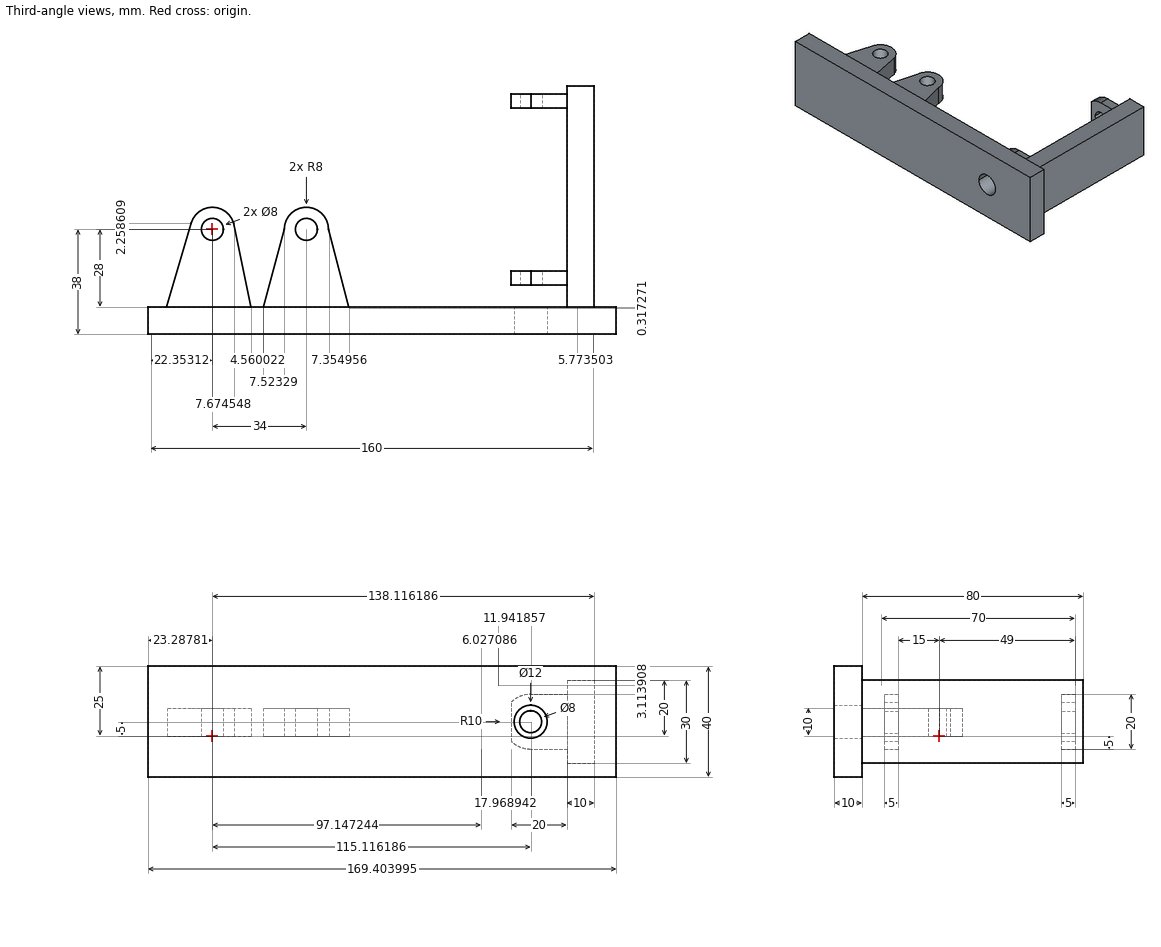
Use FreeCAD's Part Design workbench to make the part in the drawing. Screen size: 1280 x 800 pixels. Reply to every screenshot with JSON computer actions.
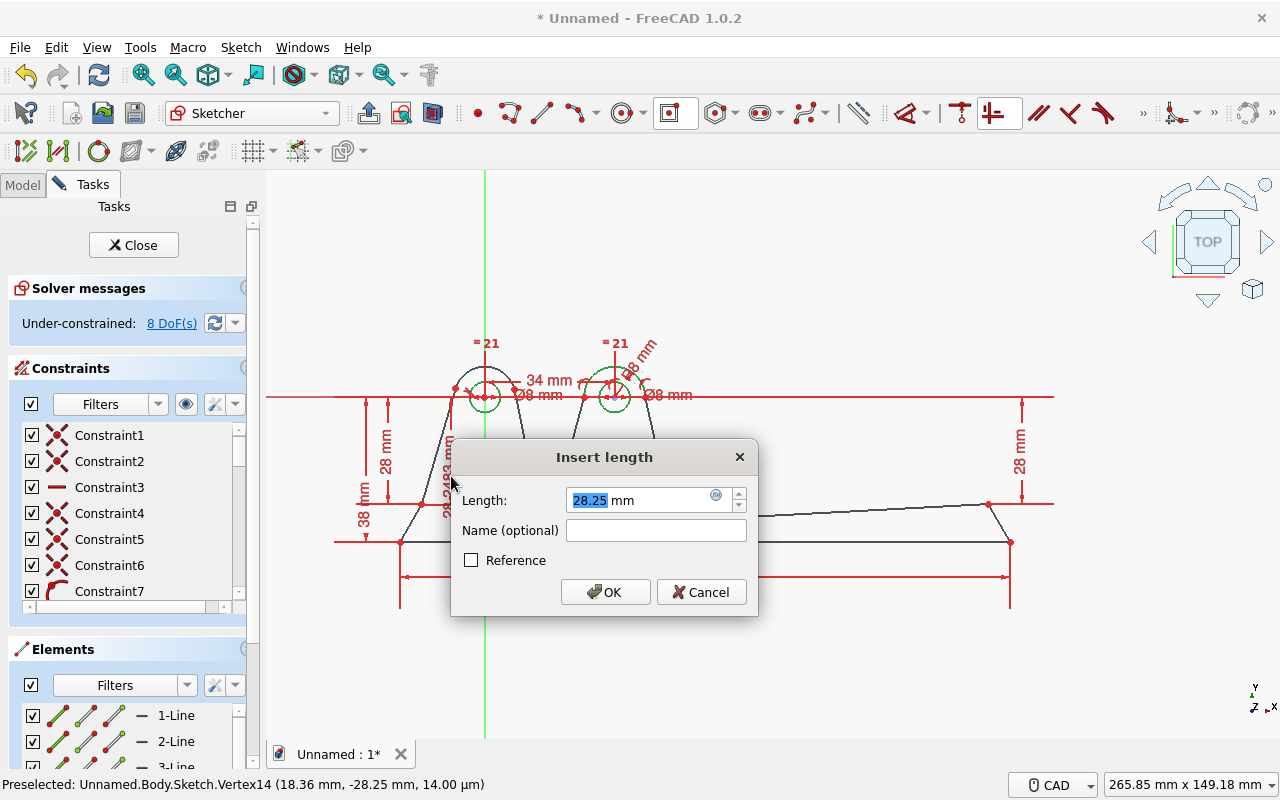
{"action": "type", "text": "28"}
{"action": "key", "text": "Return"}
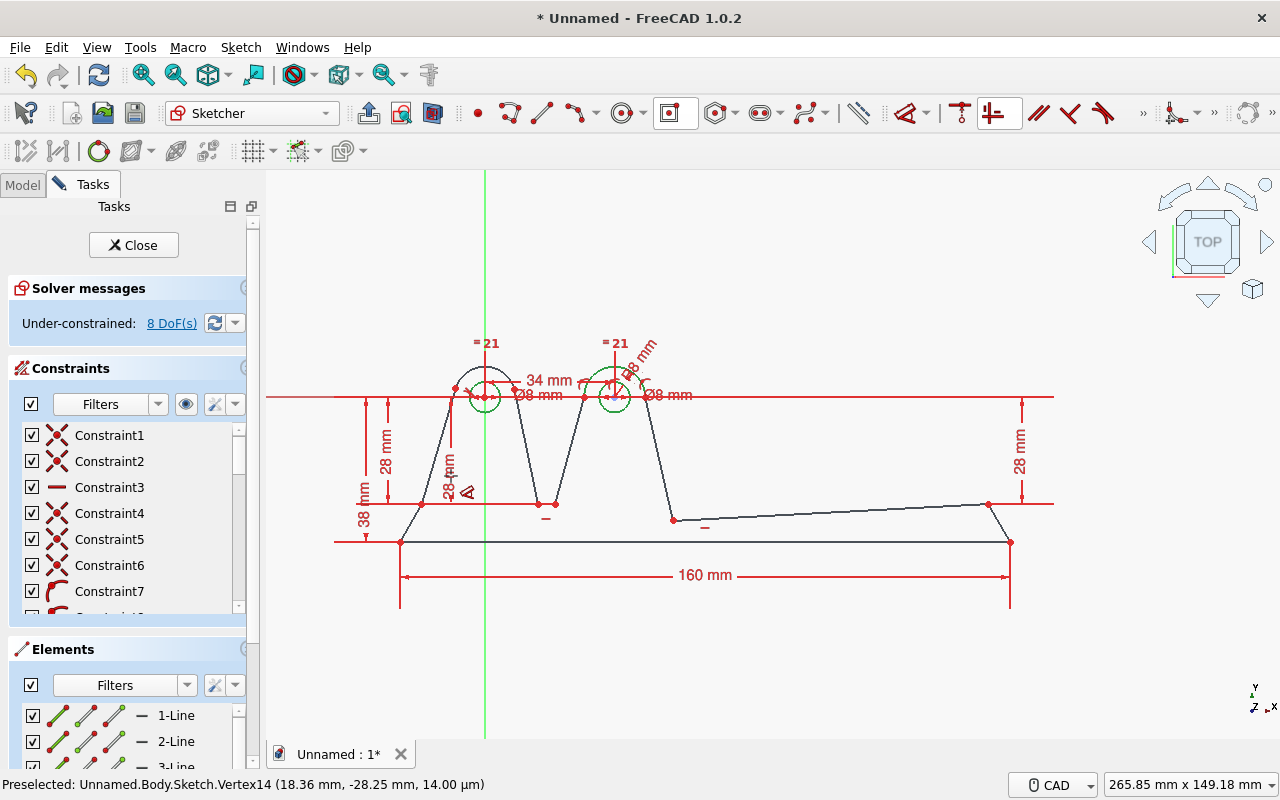
{"action": "scroll", "coordinate": [546, 504], "scroll_direction": "up", "scroll_amount": 5}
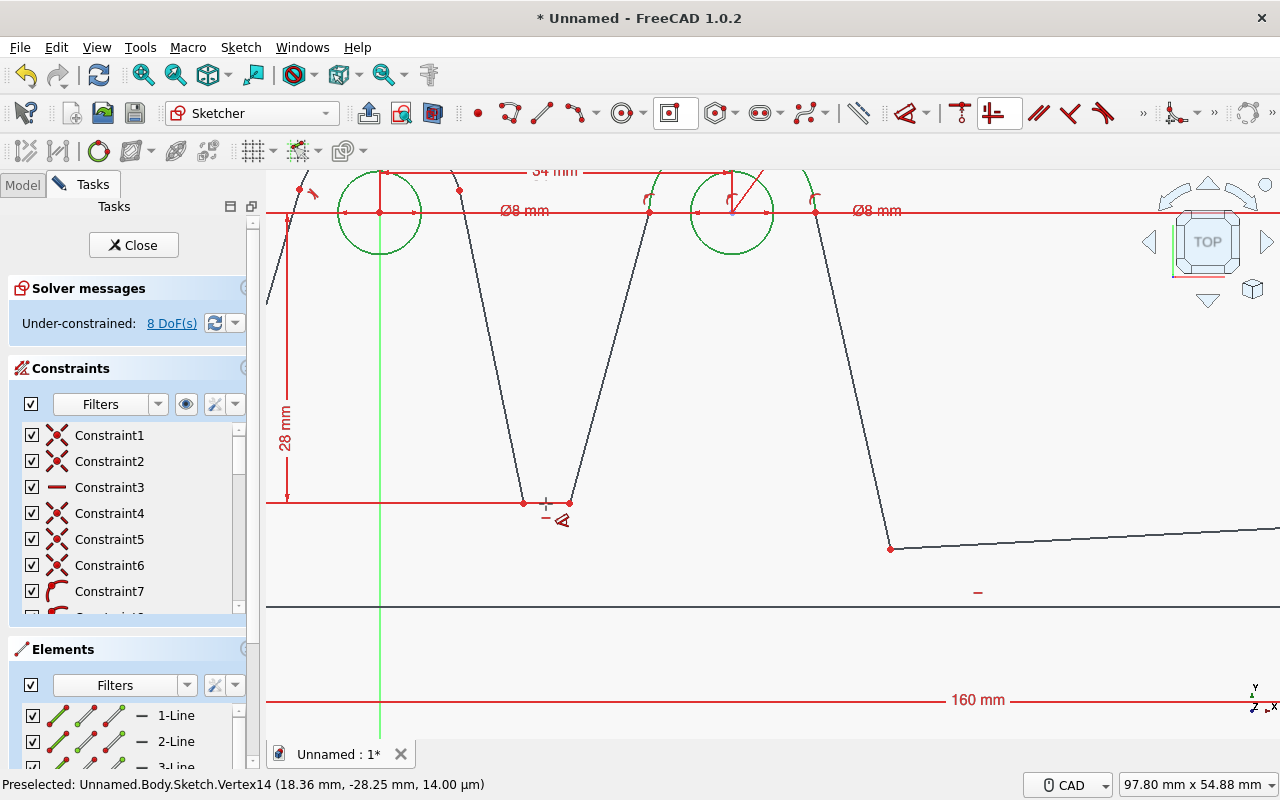
{"action": "left_click", "coordinate": [547, 503]}
{"action": "left_click", "coordinate": [547, 537]}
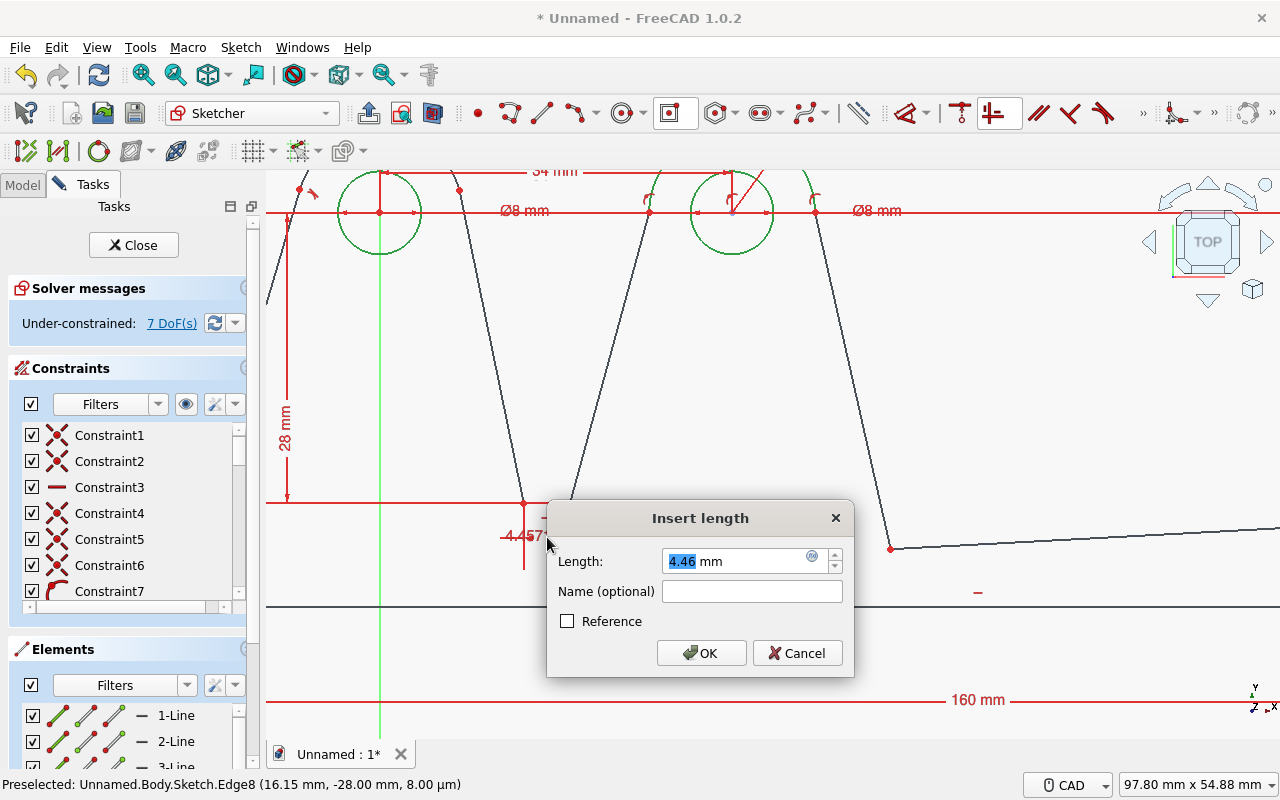
{"action": "type", "text": "4.560022"}
{"action": "key", "text": "Return"}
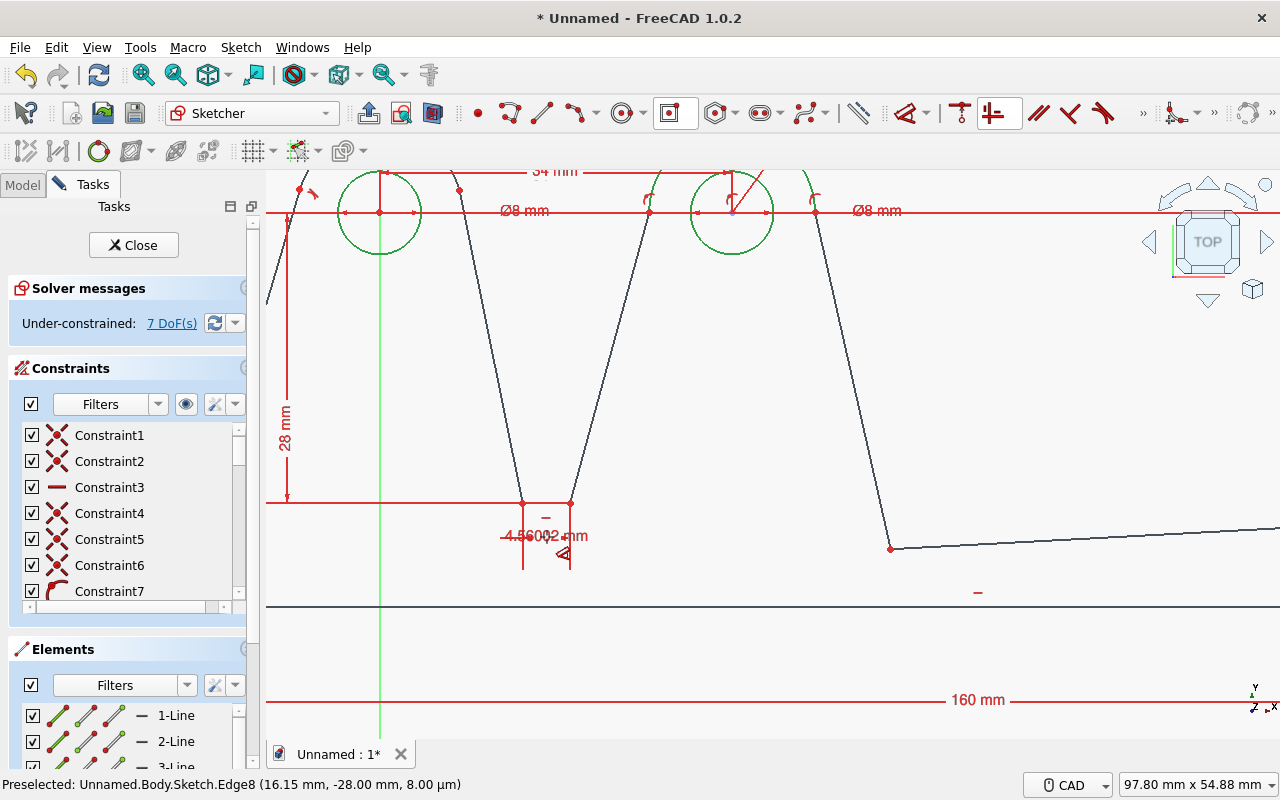
{"action": "left_click", "coordinate": [625, 300]}
{"action": "left_click", "coordinate": [628, 537]}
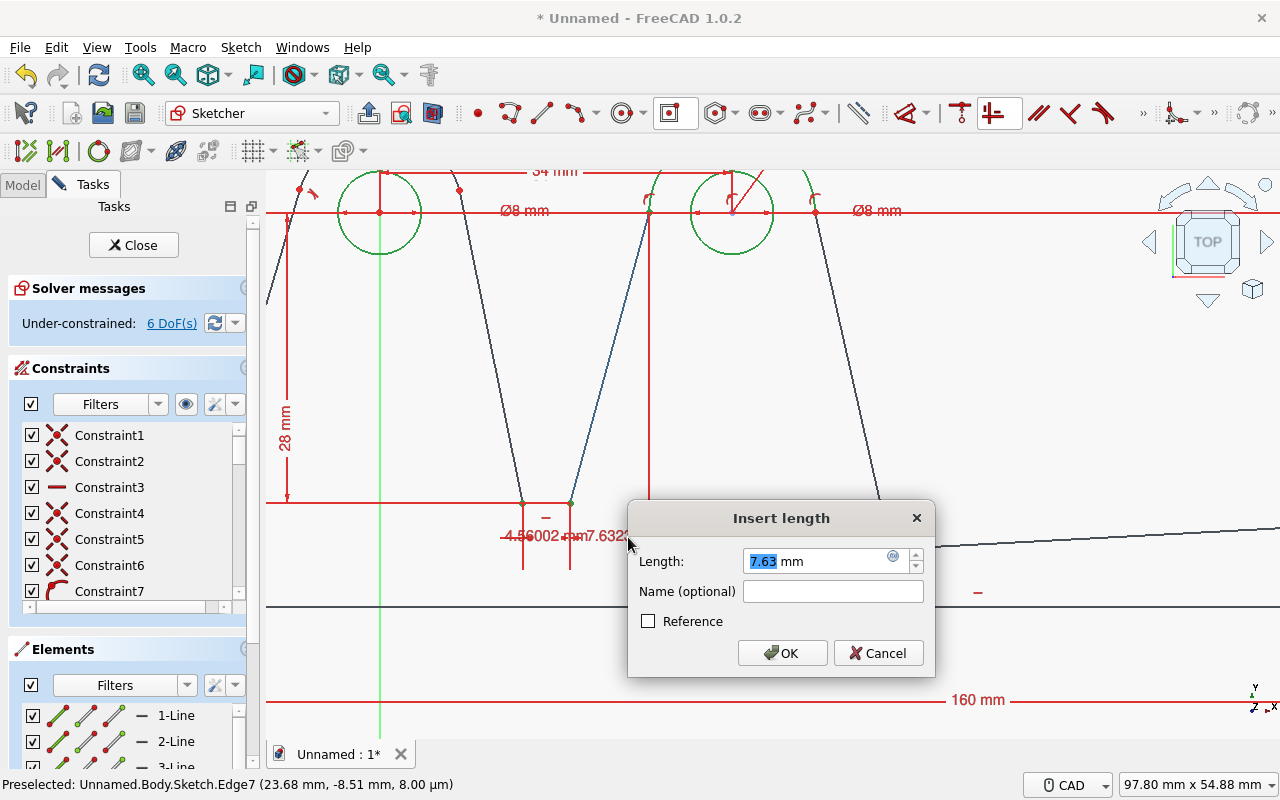
{"action": "type", "text": "7.52329"}
{"action": "key", "text": "Return"}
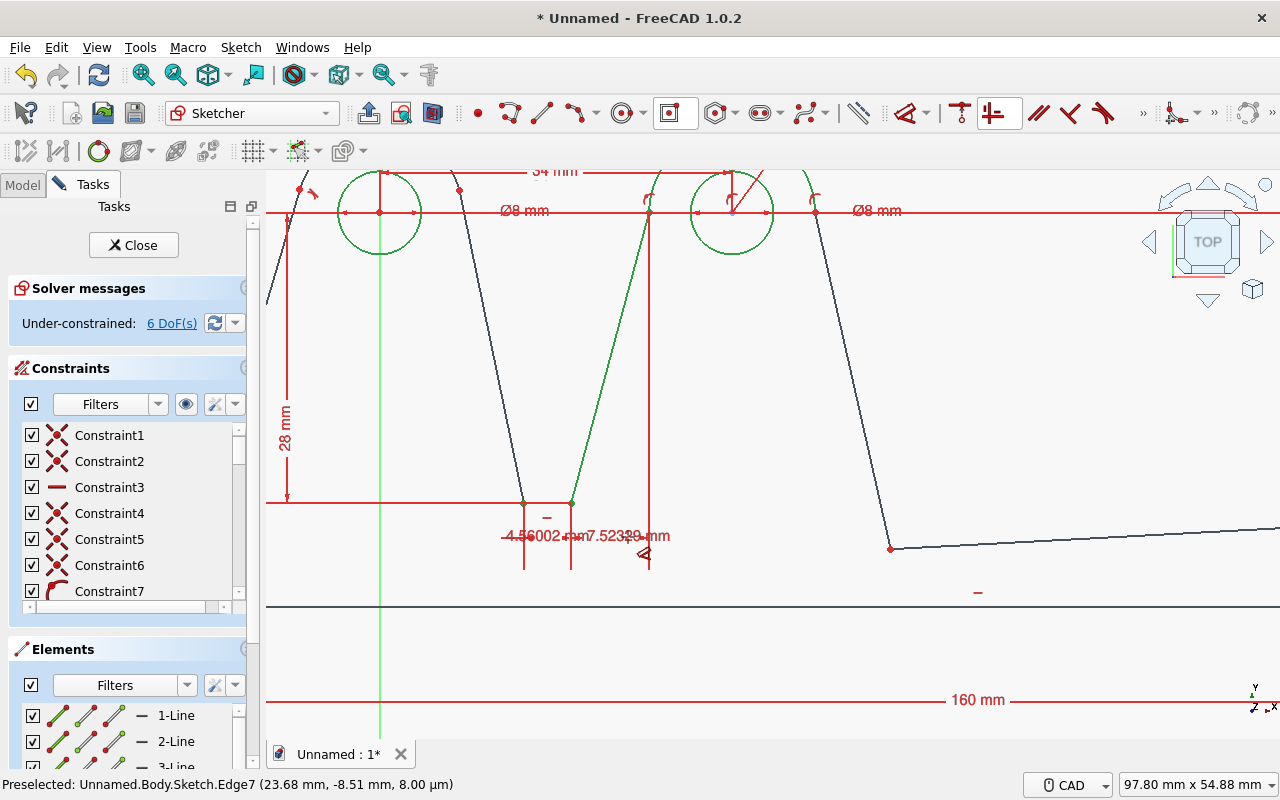
{"action": "scroll", "coordinate": [546, 505], "scroll_direction": "down", "scroll_amount": 5}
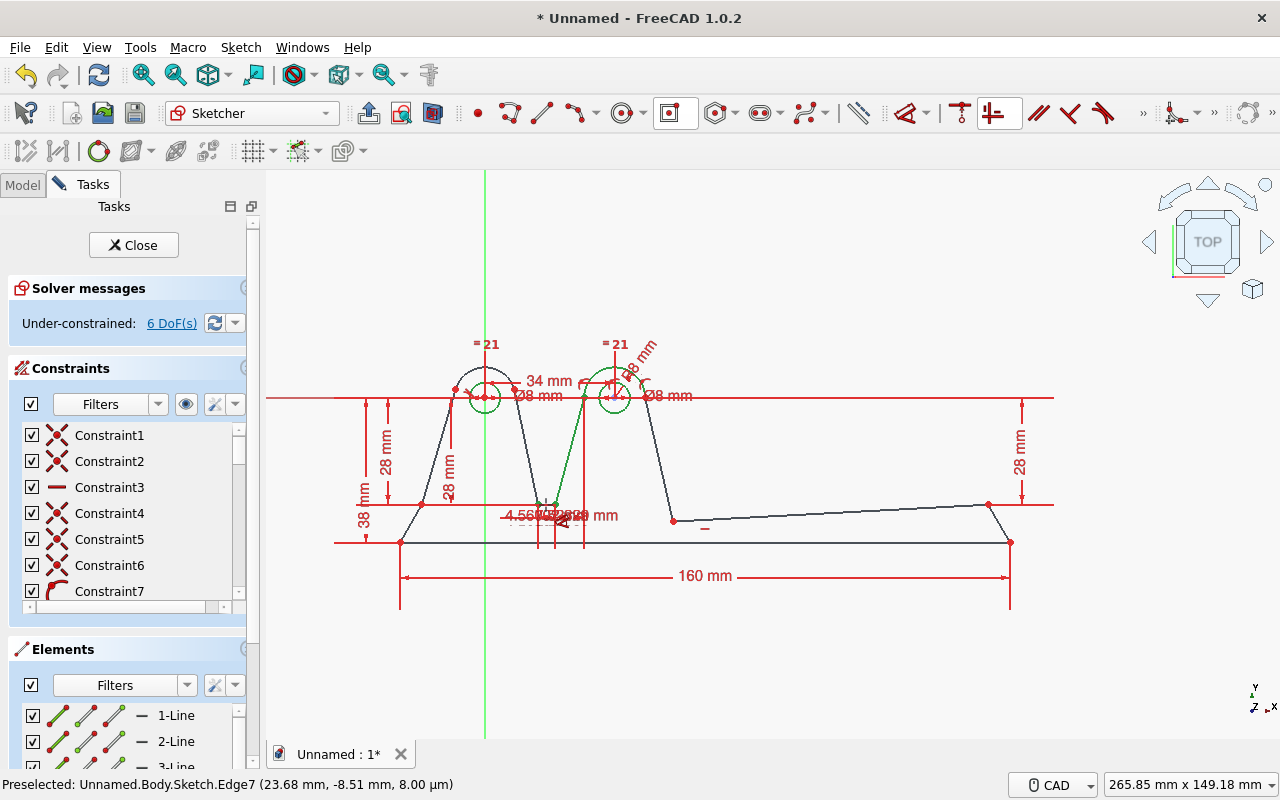
{"action": "scroll", "coordinate": [456, 389], "scroll_direction": "up", "scroll_amount": 8}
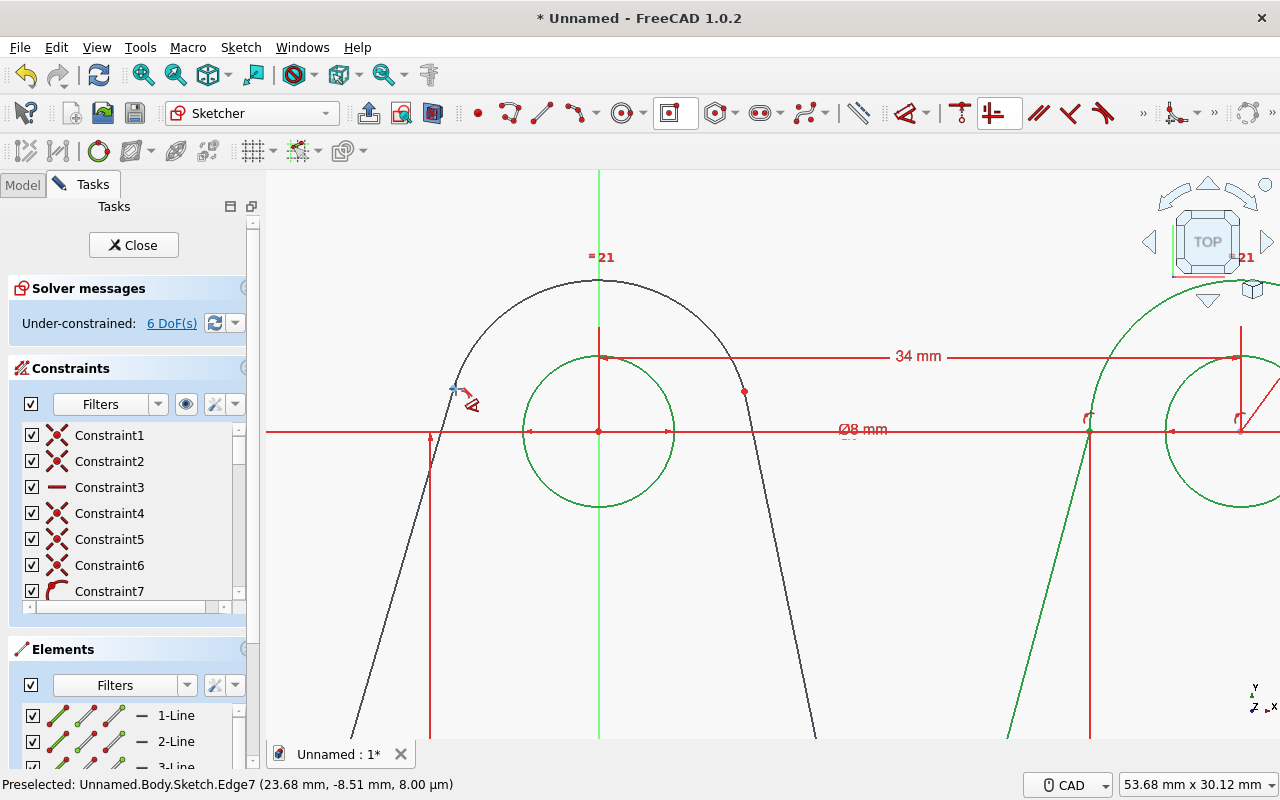
{"action": "left_click", "coordinate": [454, 389]}
{"action": "left_click", "coordinate": [420, 410]}